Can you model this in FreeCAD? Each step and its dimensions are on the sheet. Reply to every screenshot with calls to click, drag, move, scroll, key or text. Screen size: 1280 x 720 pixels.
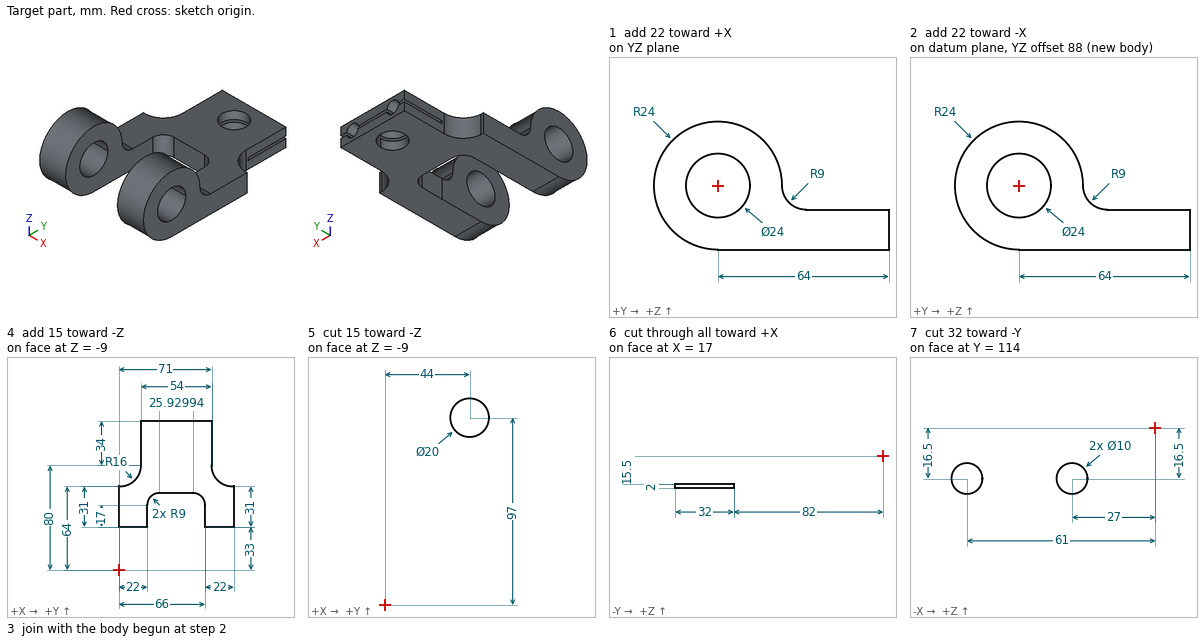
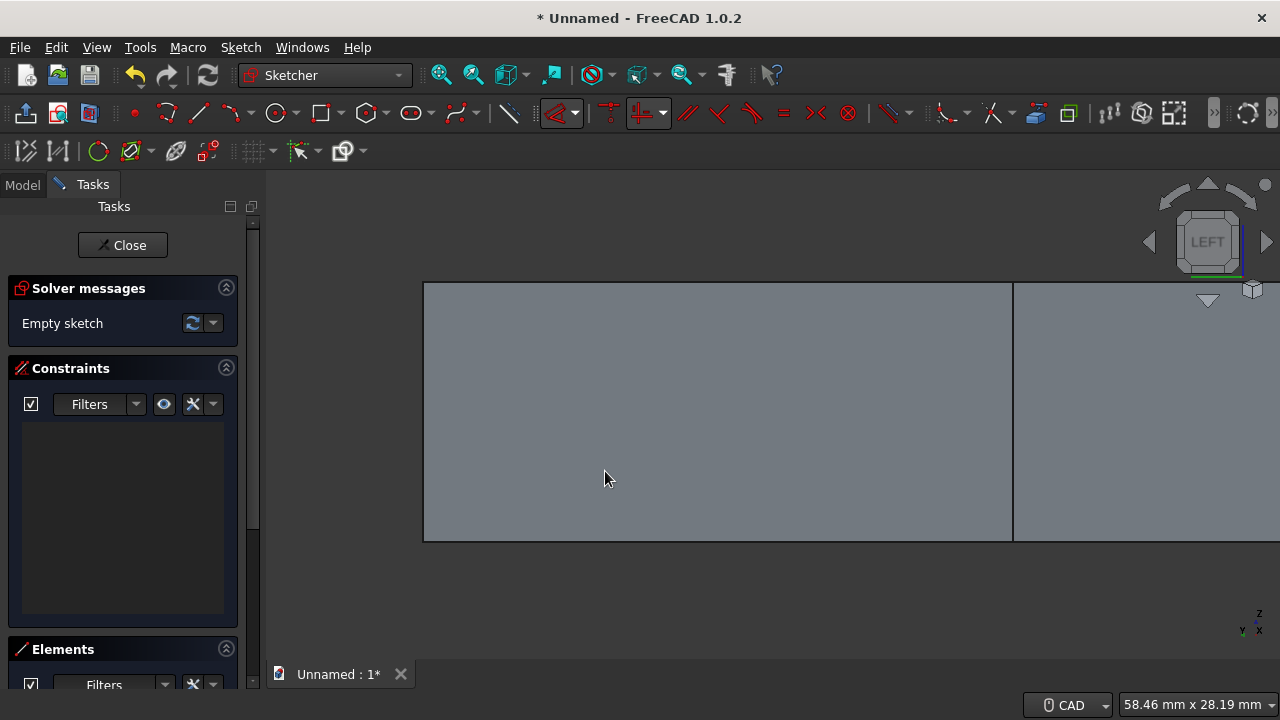
click(322, 114)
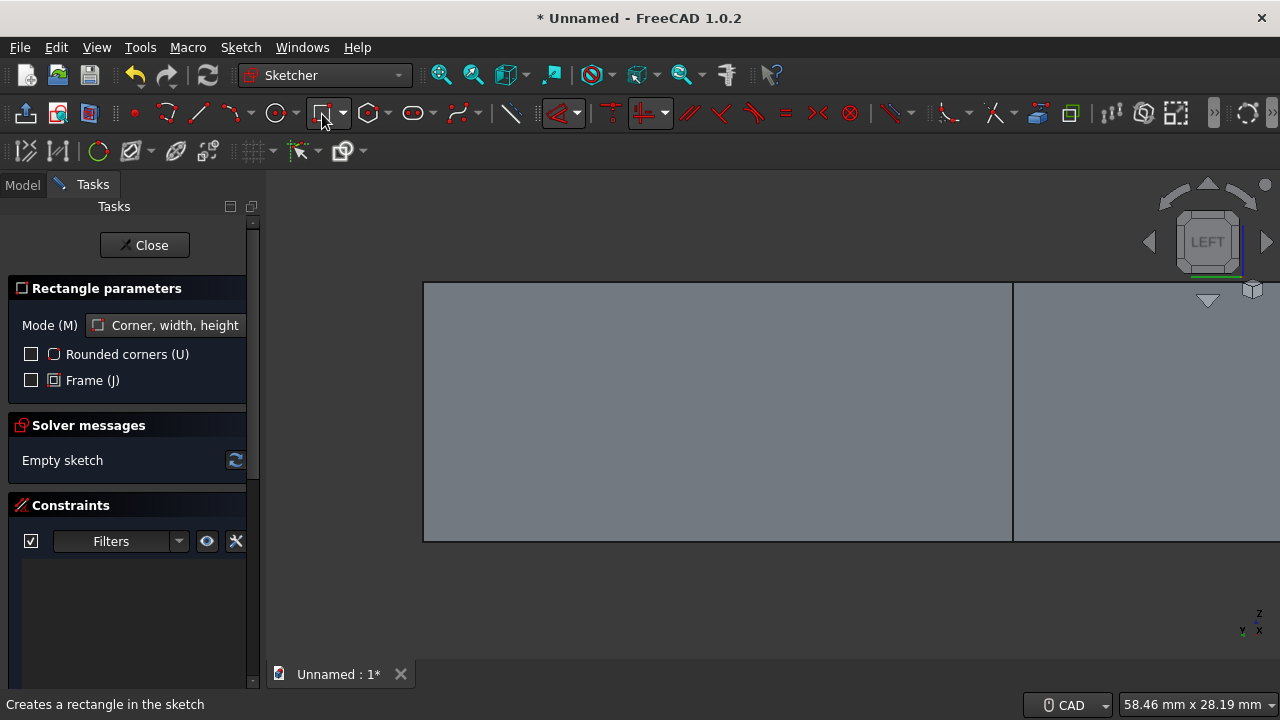
click(423, 395)
click(978, 430)
key(Escape)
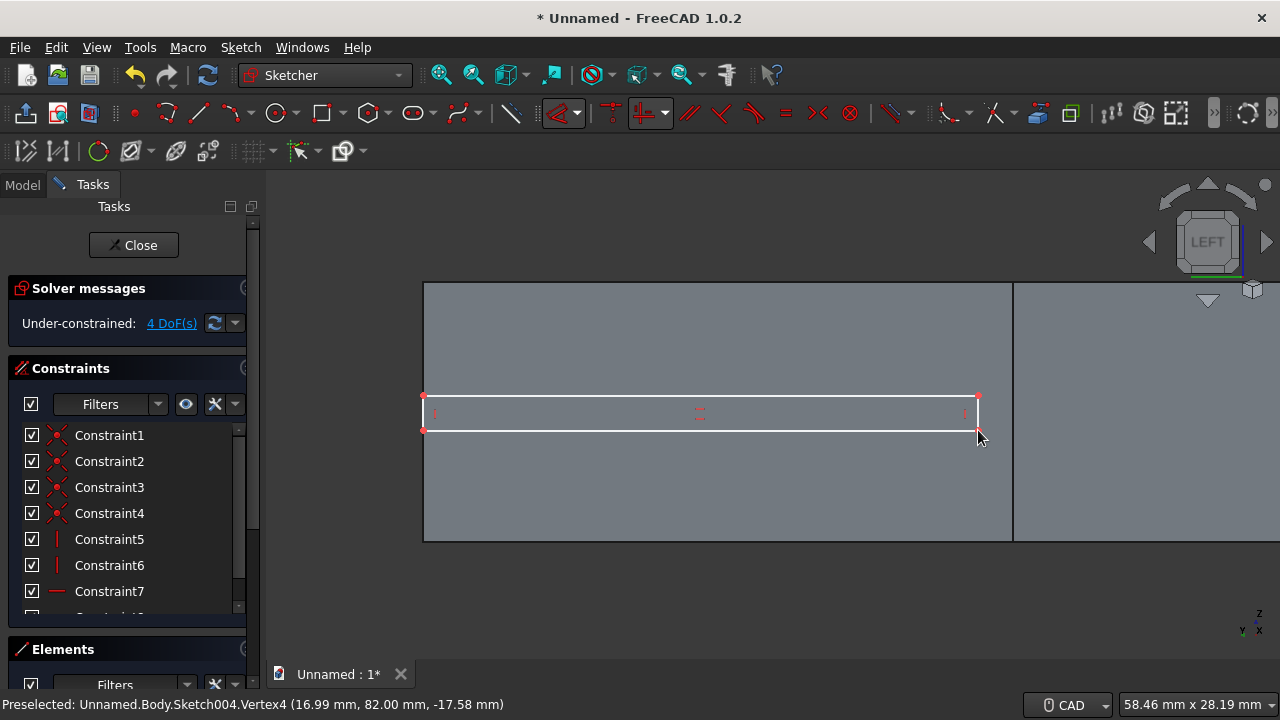
scroll(423, 406, up, 2)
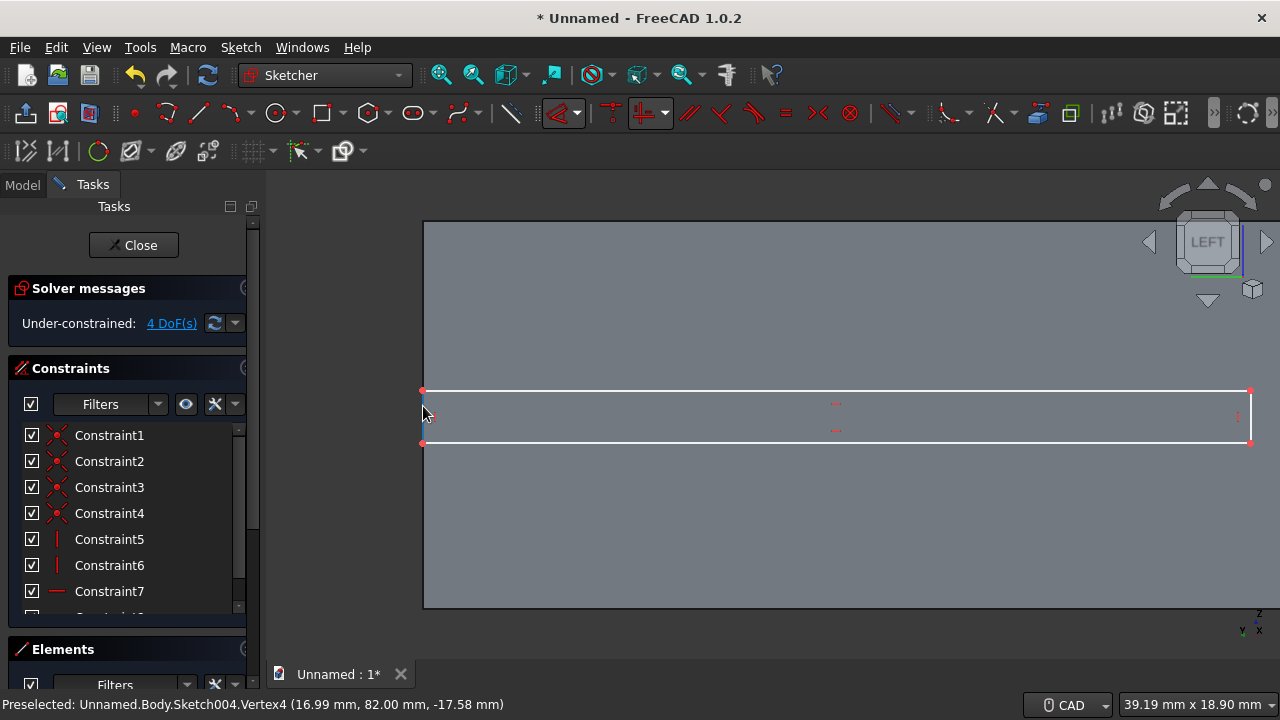
click(423, 407)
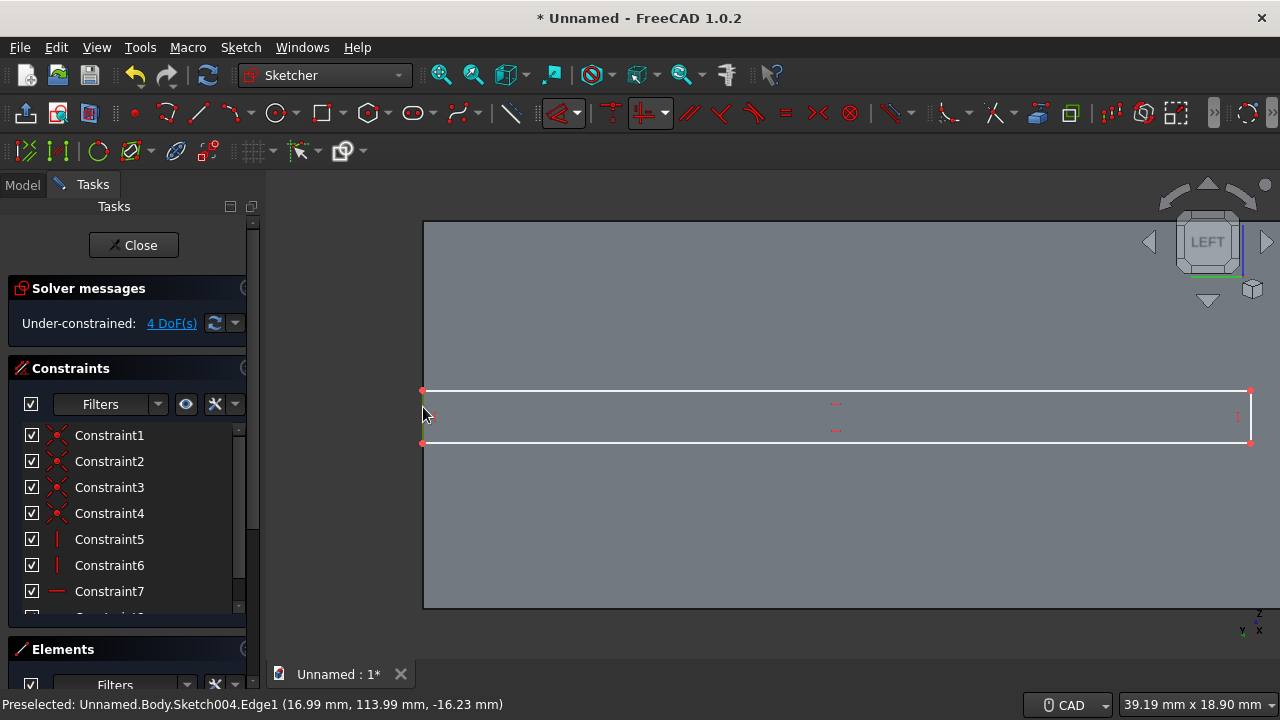
click(580, 114)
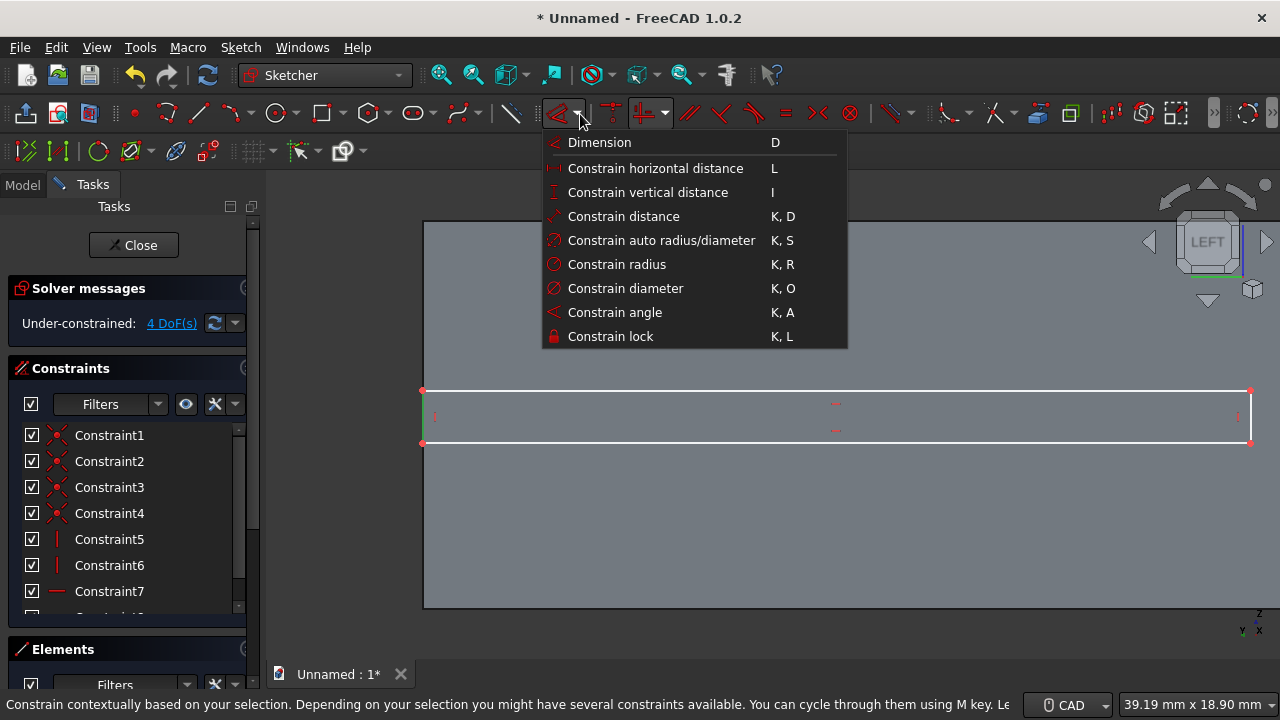
click(695, 192)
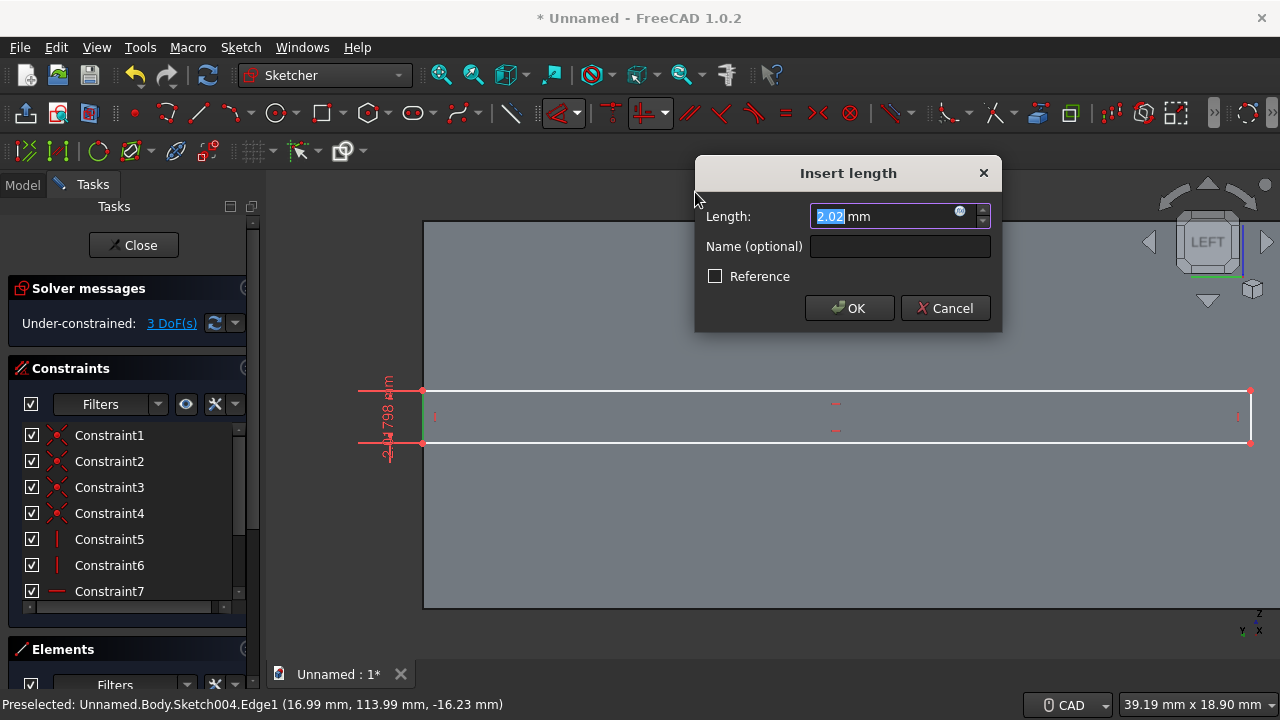
text(2)
key(Return)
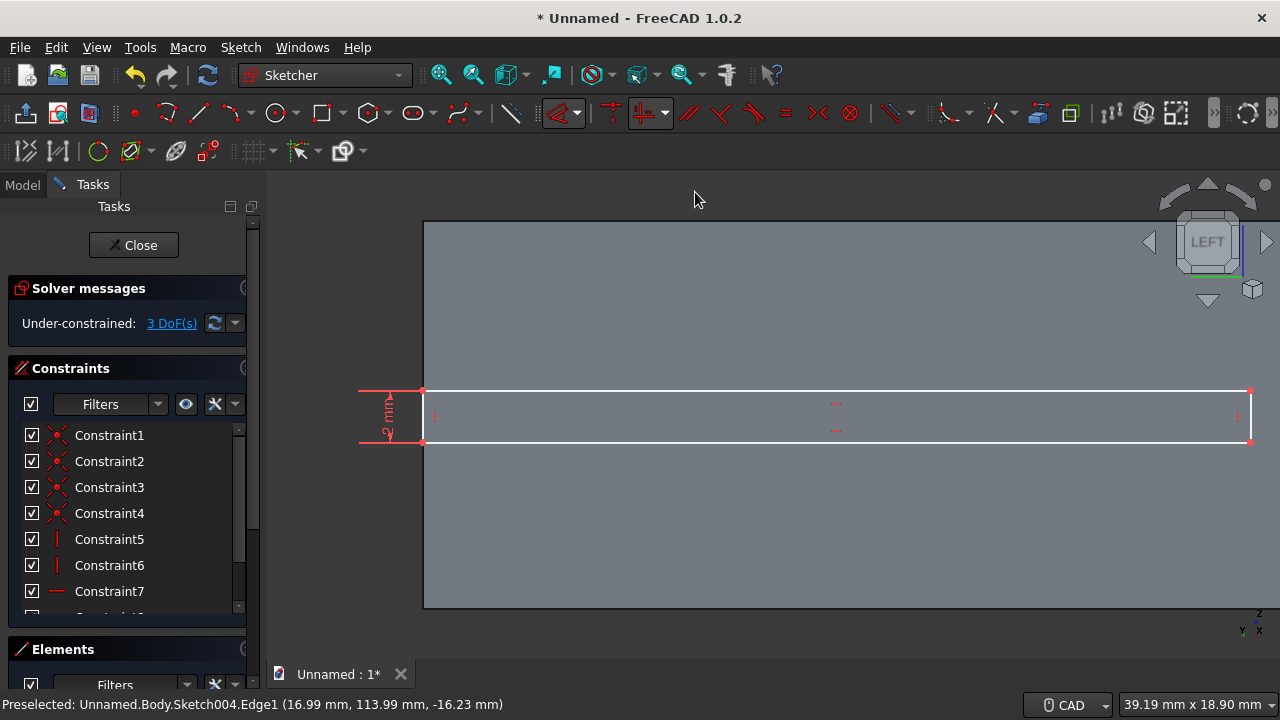
click(671, 443)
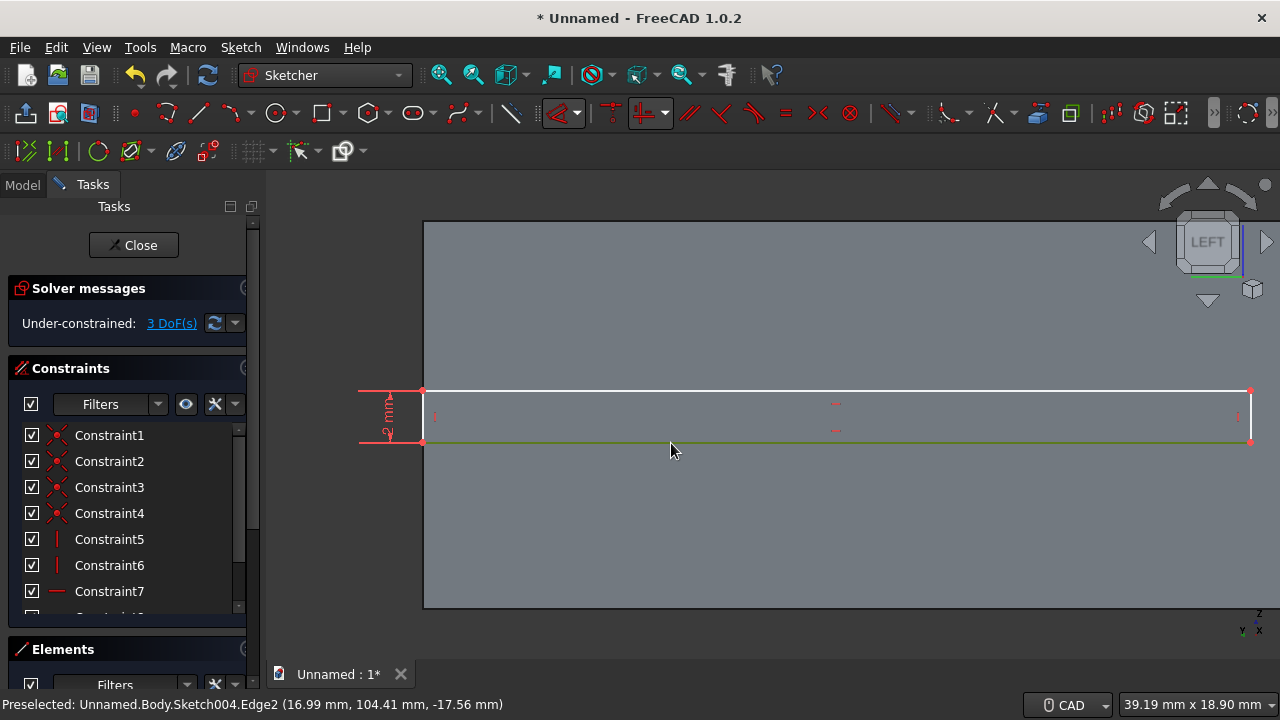
key(l)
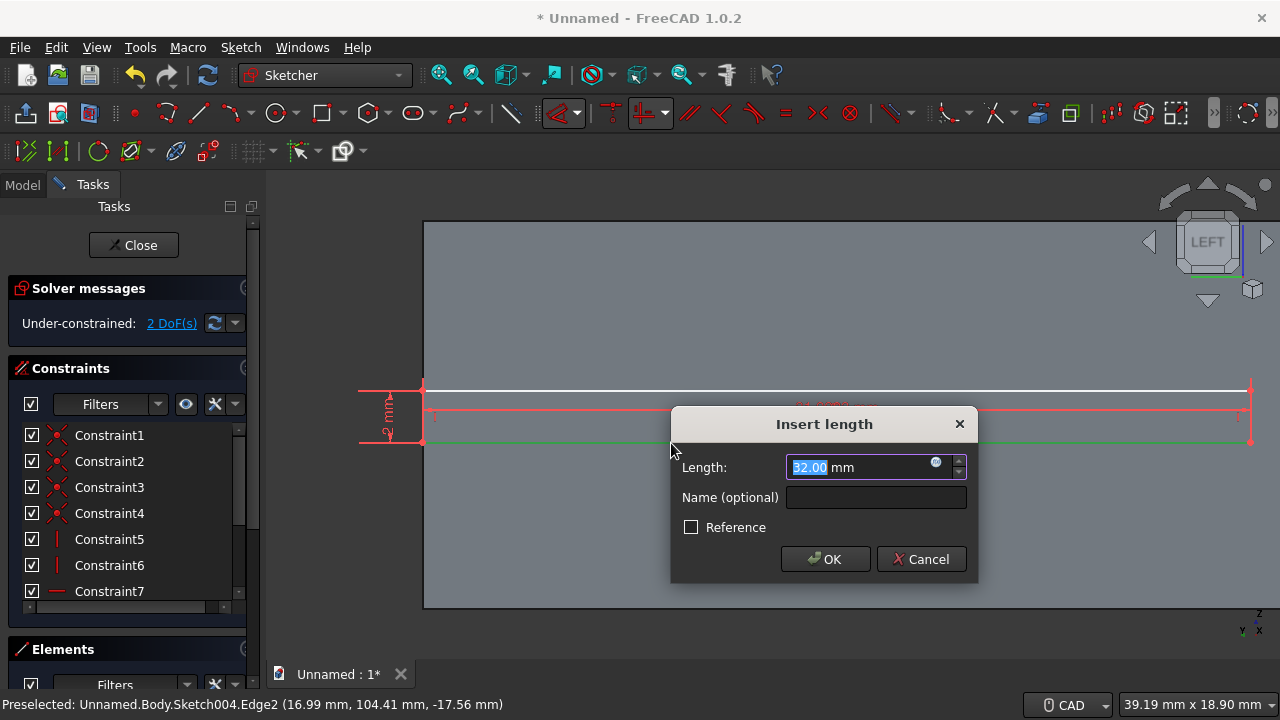
text(32)
key(Return)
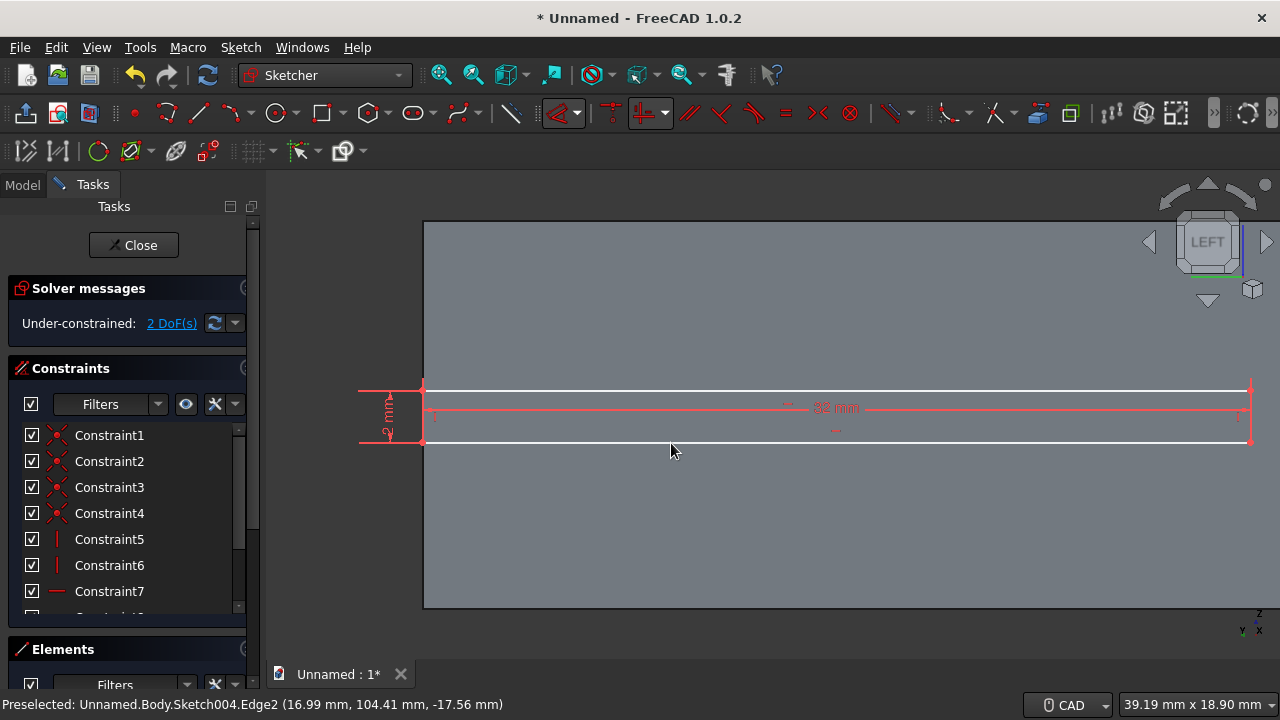
scroll(436, 413, down, 2)